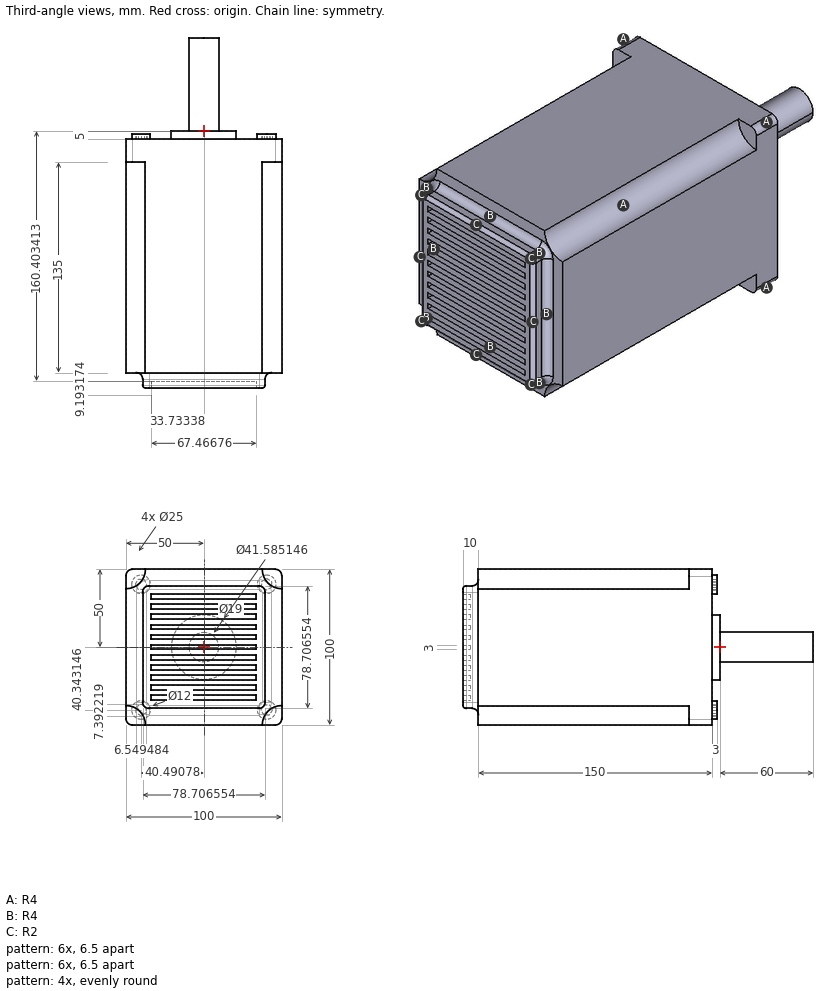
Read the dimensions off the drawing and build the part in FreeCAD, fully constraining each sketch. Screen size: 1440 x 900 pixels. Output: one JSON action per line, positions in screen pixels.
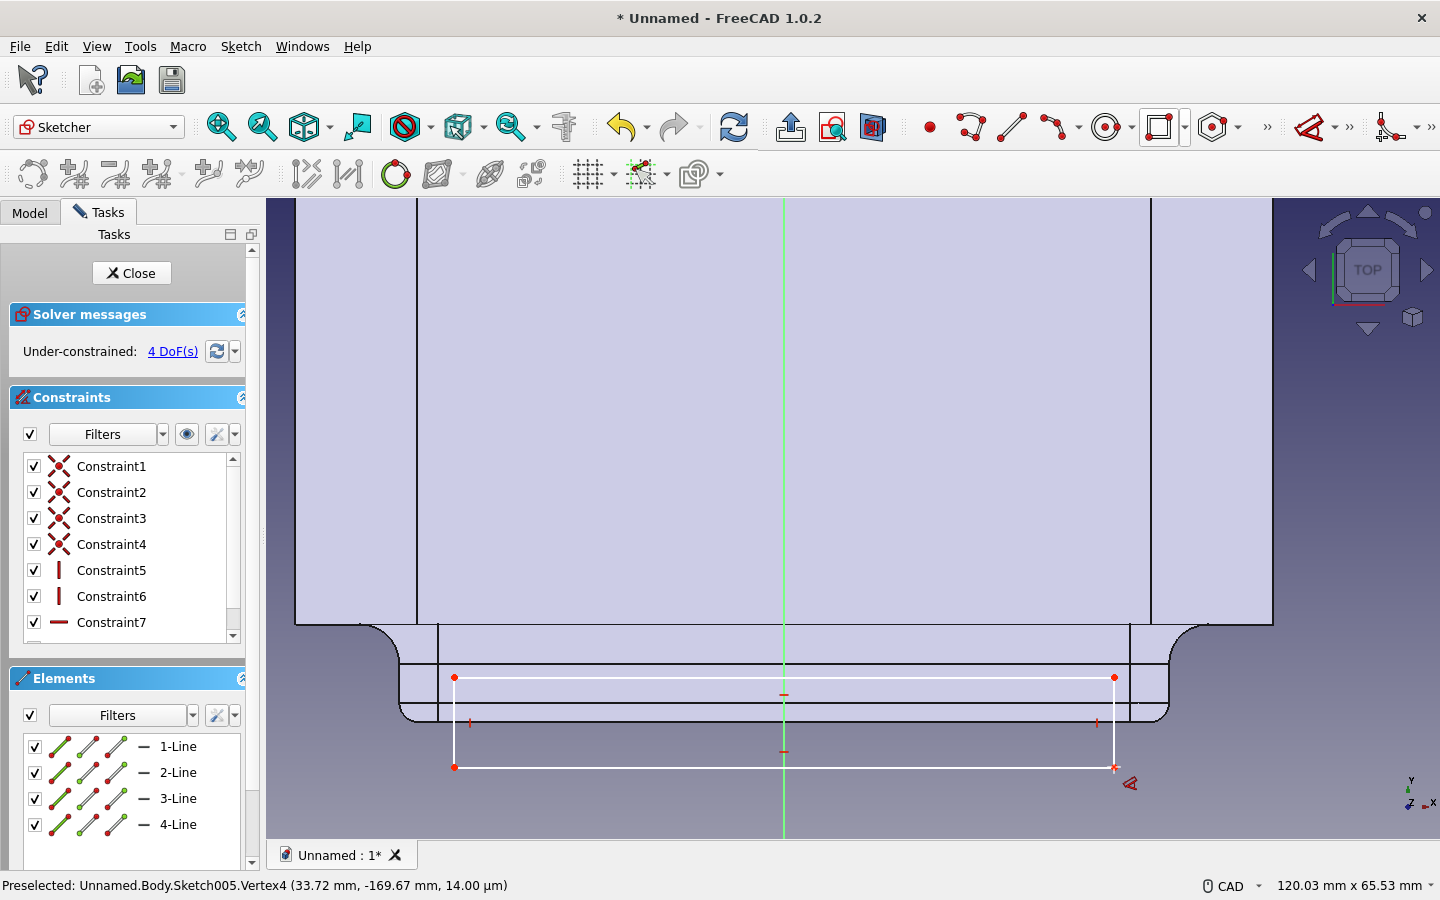
{"action": "left_click", "coordinate": [454, 705]}
{"action": "left_click", "coordinate": [420, 723]}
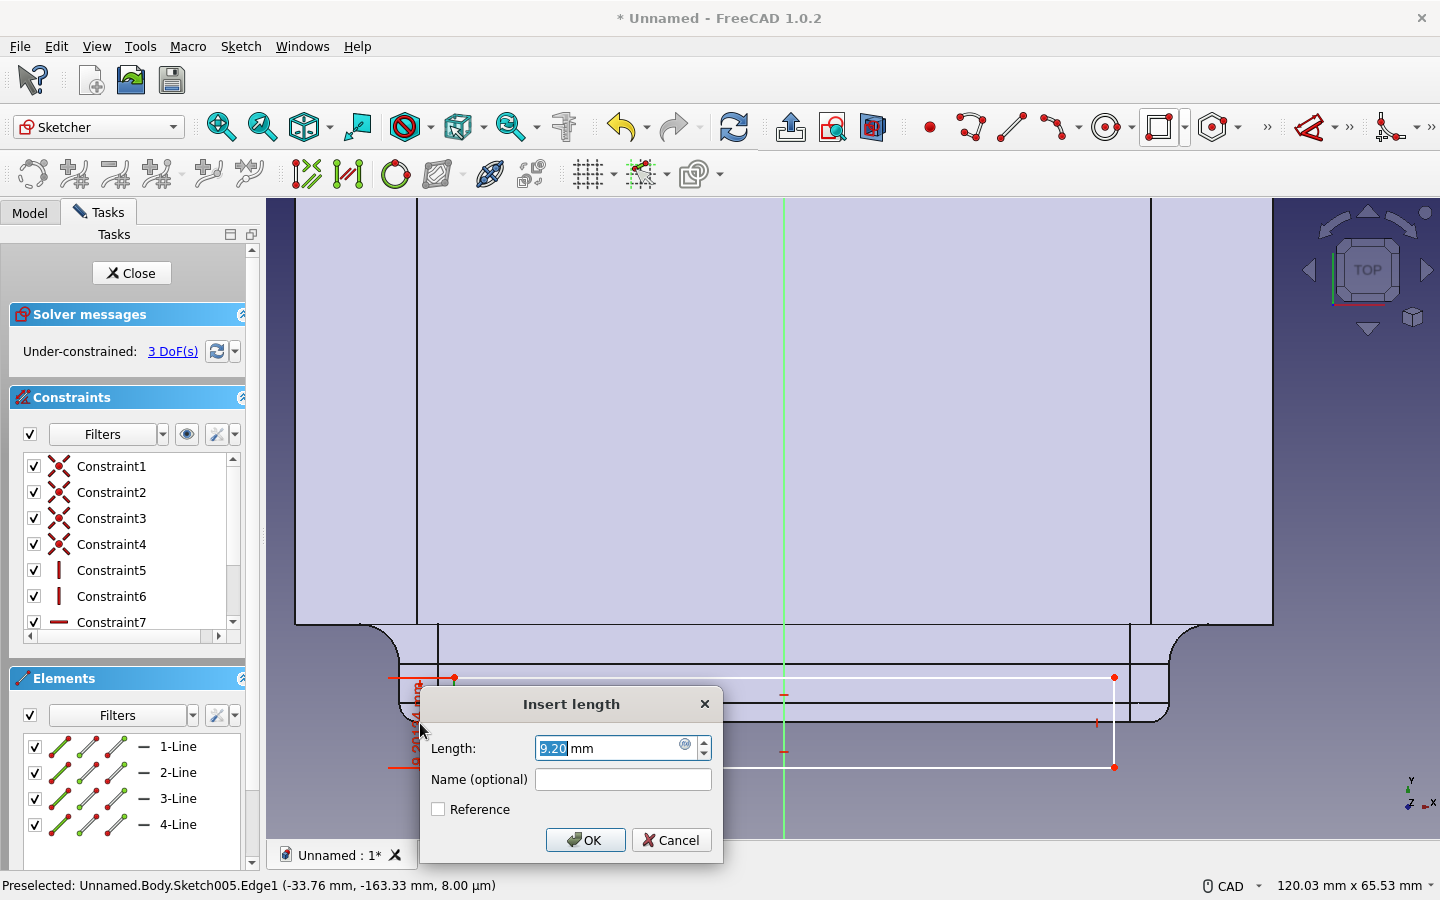
{"action": "type", "text": "9.193174"}
{"action": "key", "text": "Return"}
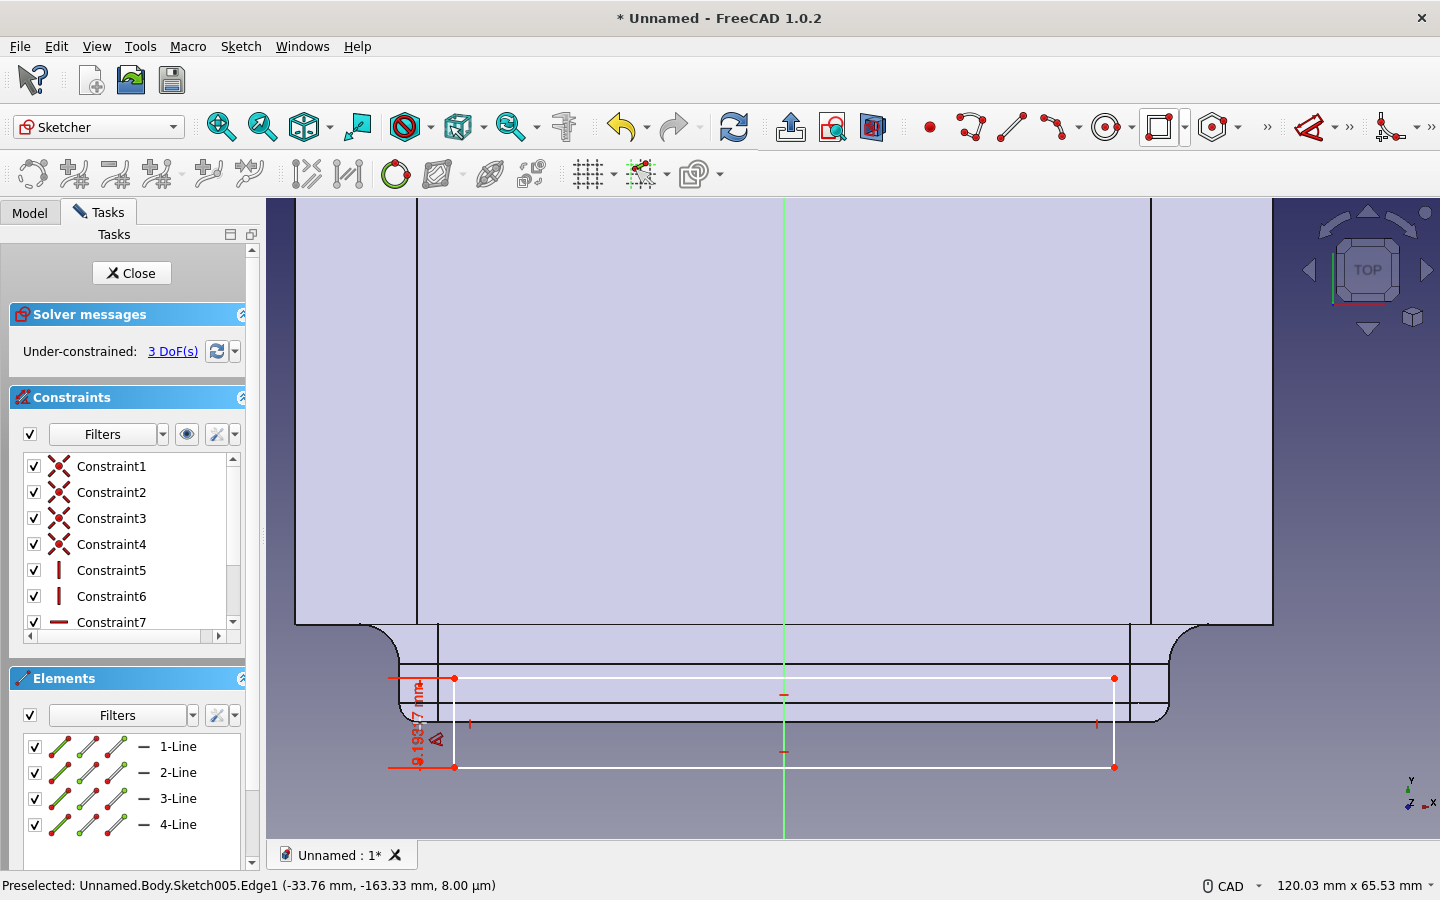
{"action": "left_click", "coordinate": [652, 768]}
{"action": "left_click", "coordinate": [632, 802]}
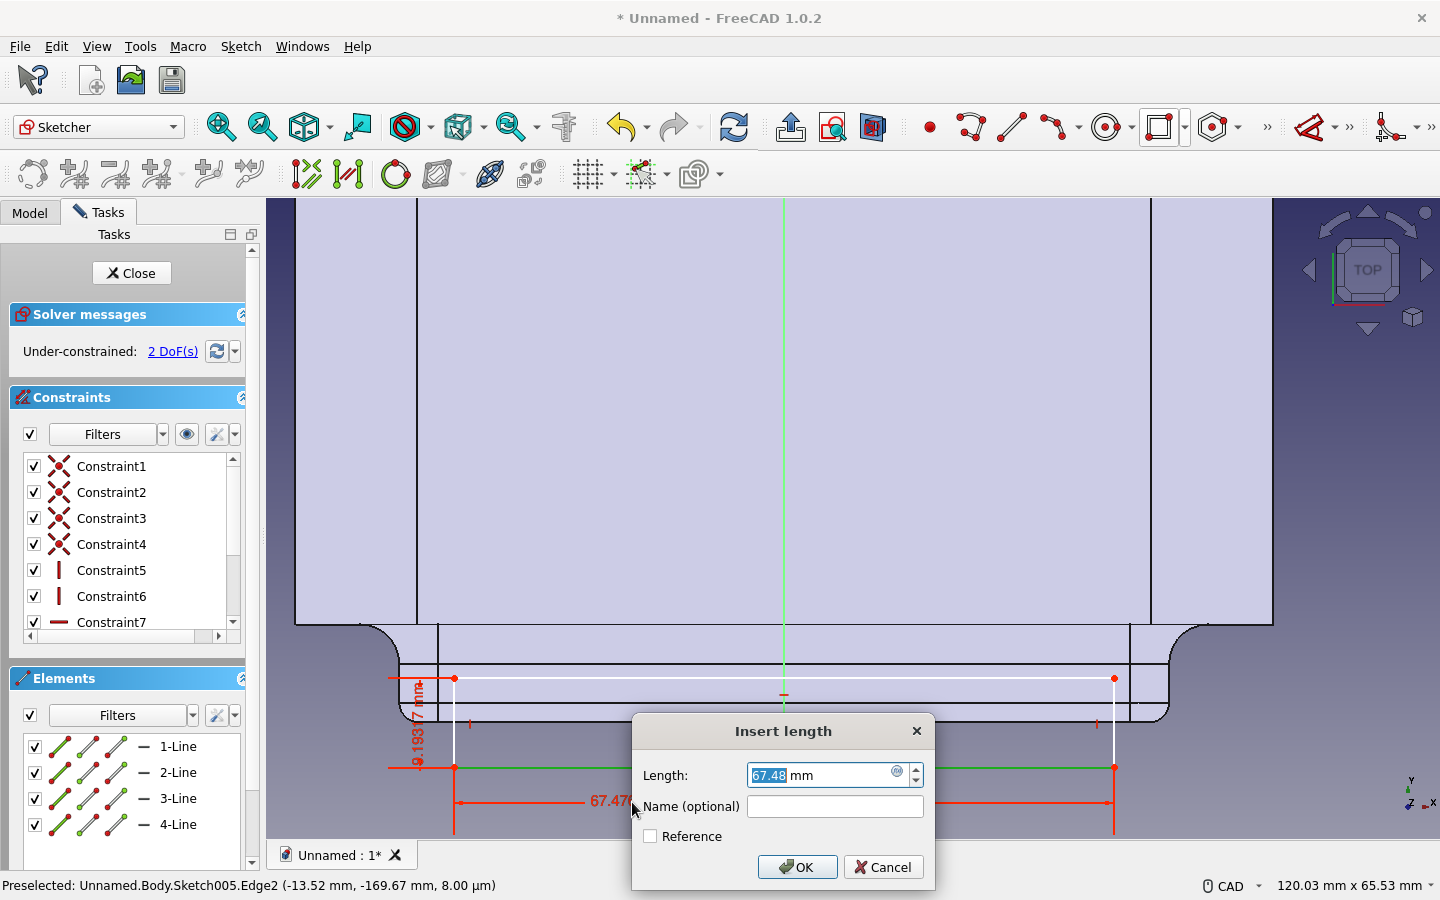
{"action": "type", "text": "67.46676"}
{"action": "key", "text": "Return"}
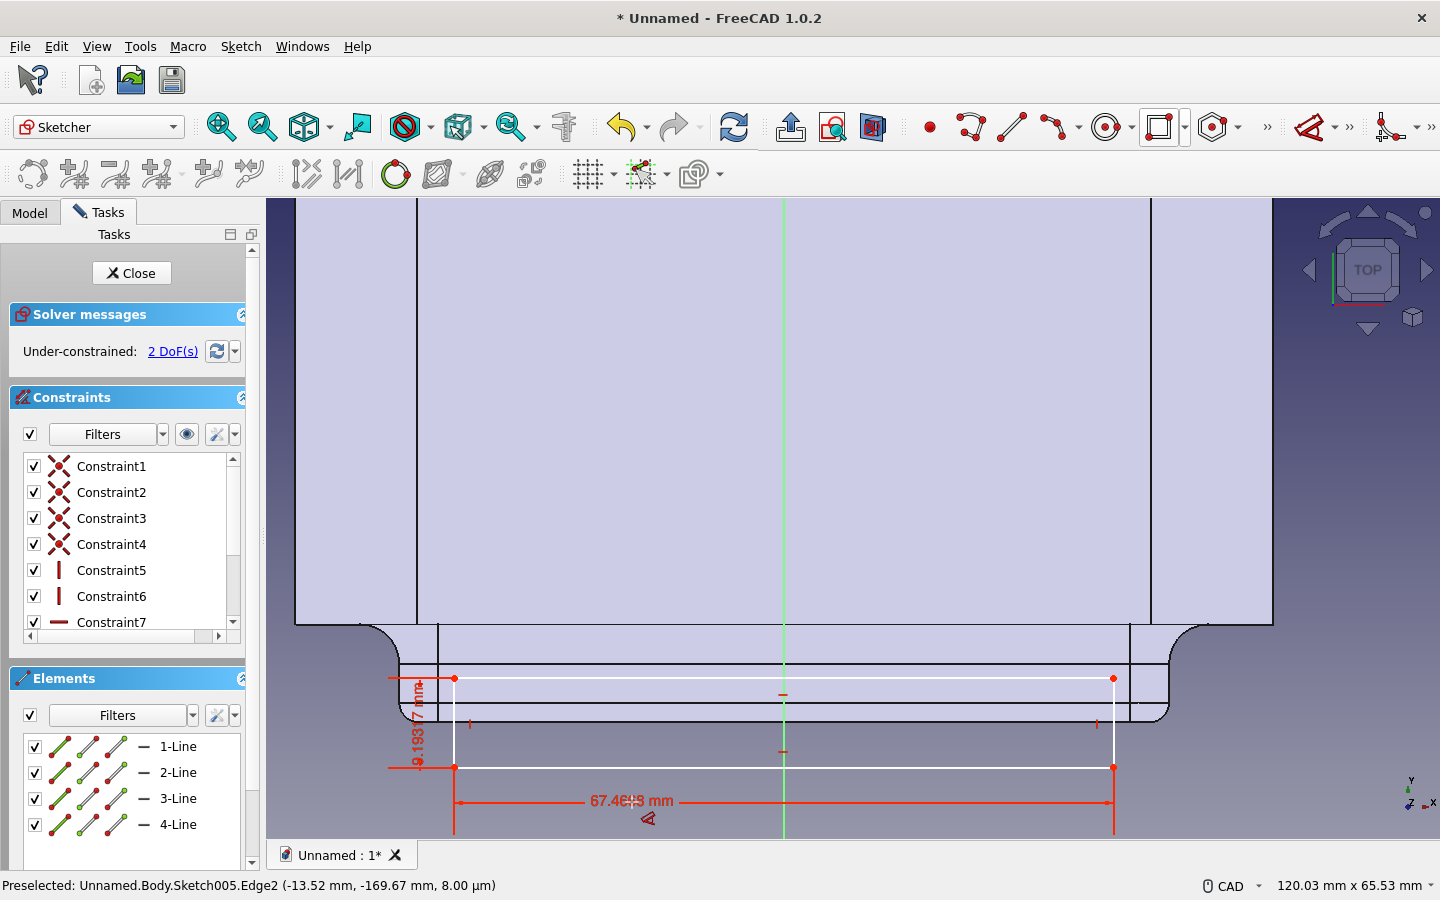
{"action": "left_click", "coordinate": [454, 678]}
{"action": "left_click", "coordinate": [619, 712]}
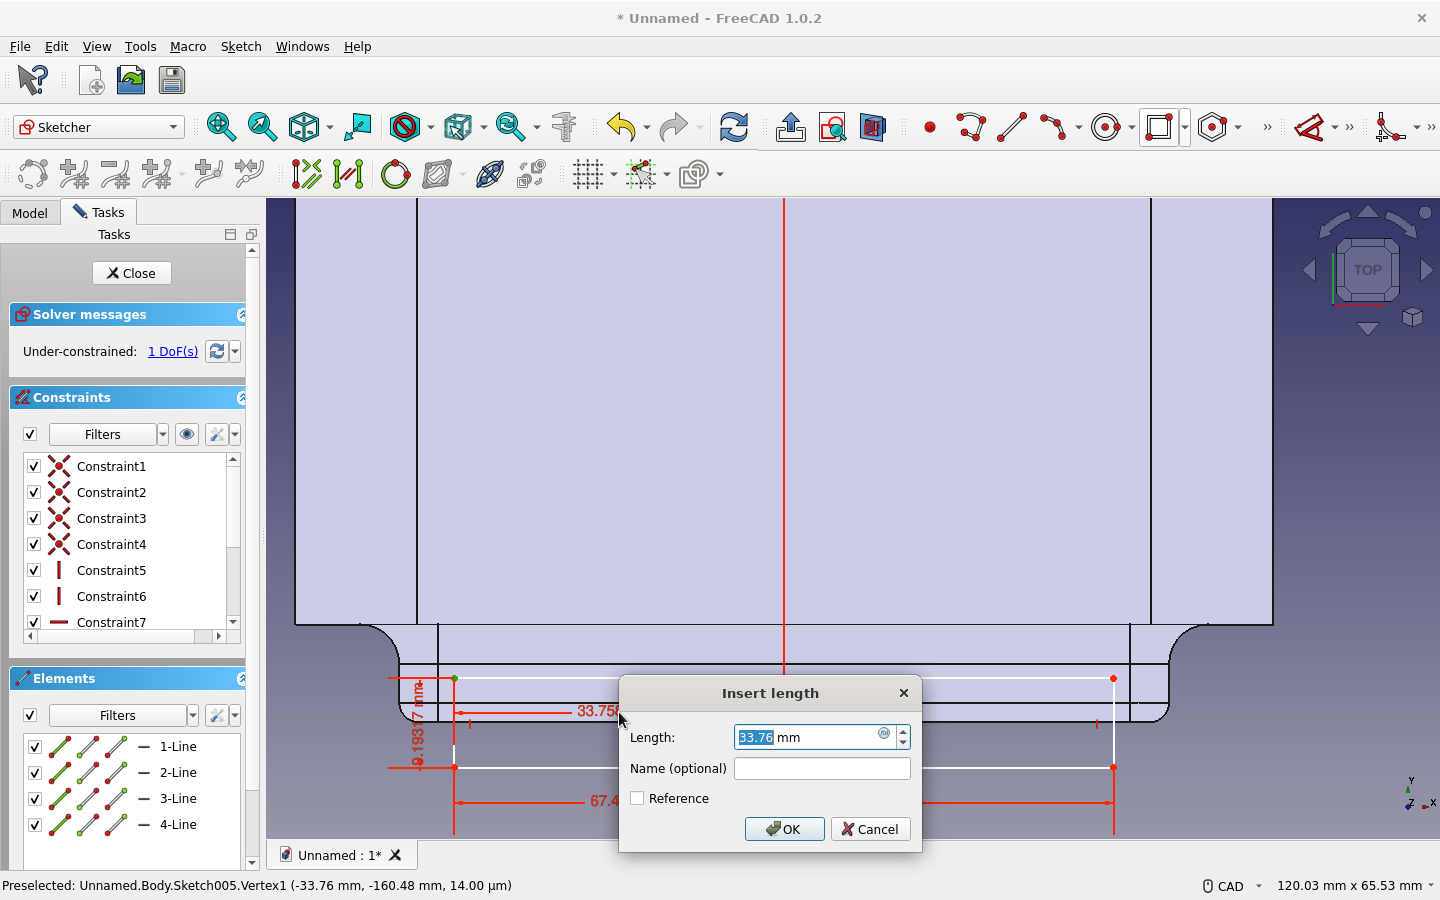
{"action": "type", "text": "33.73338"}
{"action": "key", "text": "Return"}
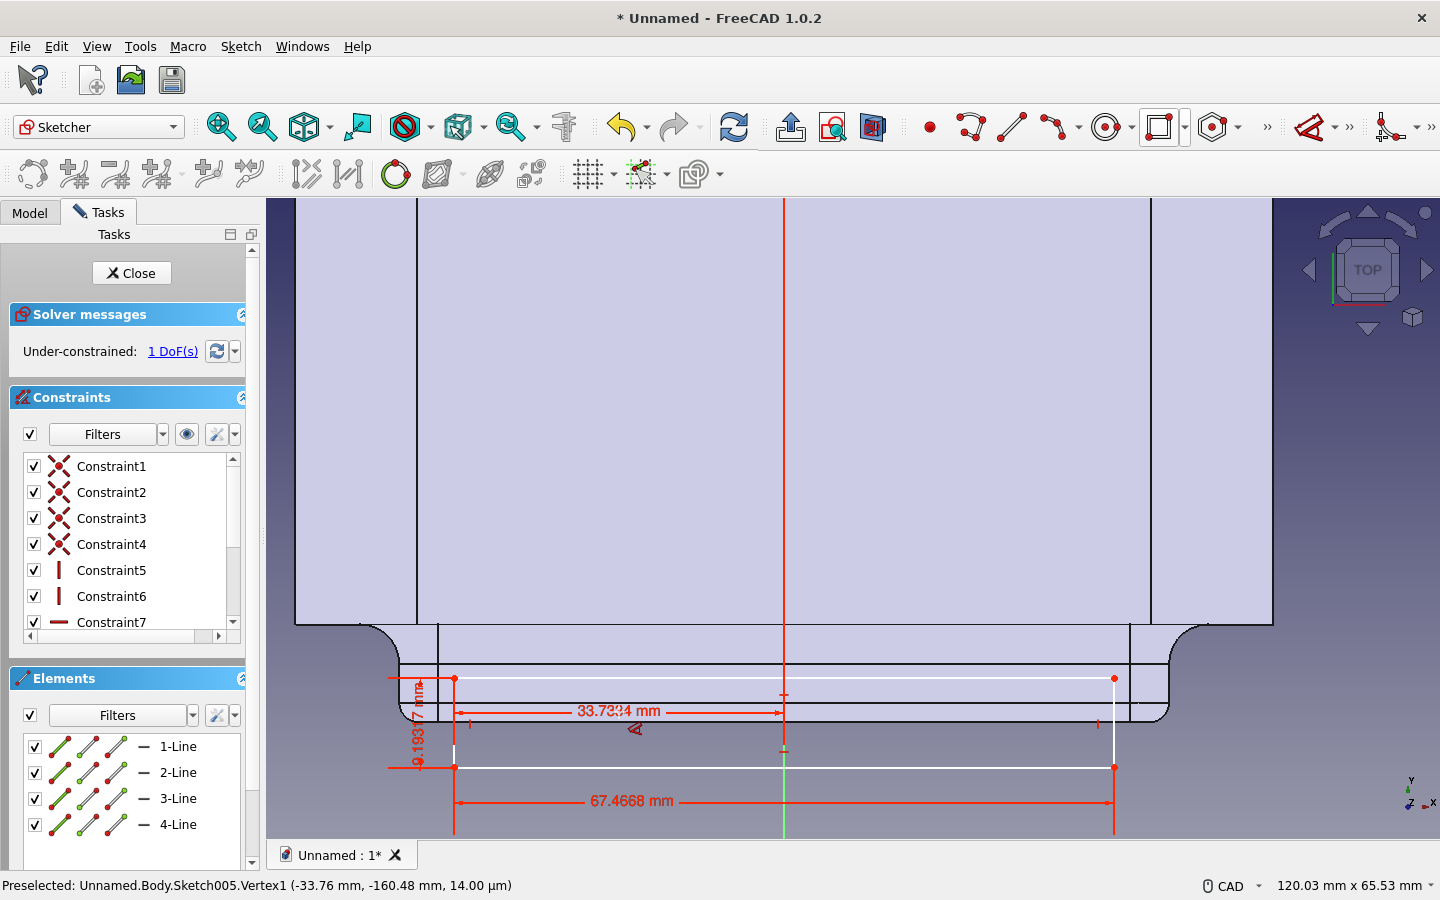
{"action": "left_click", "coordinate": [454, 678]}
{"action": "left_click", "coordinate": [420, 452]}